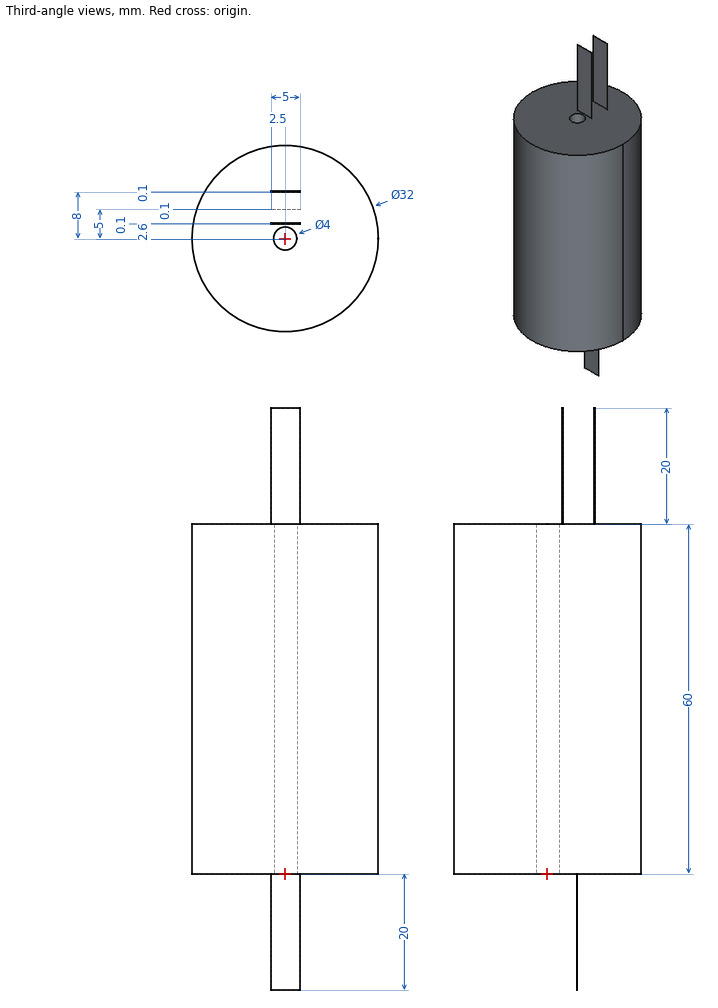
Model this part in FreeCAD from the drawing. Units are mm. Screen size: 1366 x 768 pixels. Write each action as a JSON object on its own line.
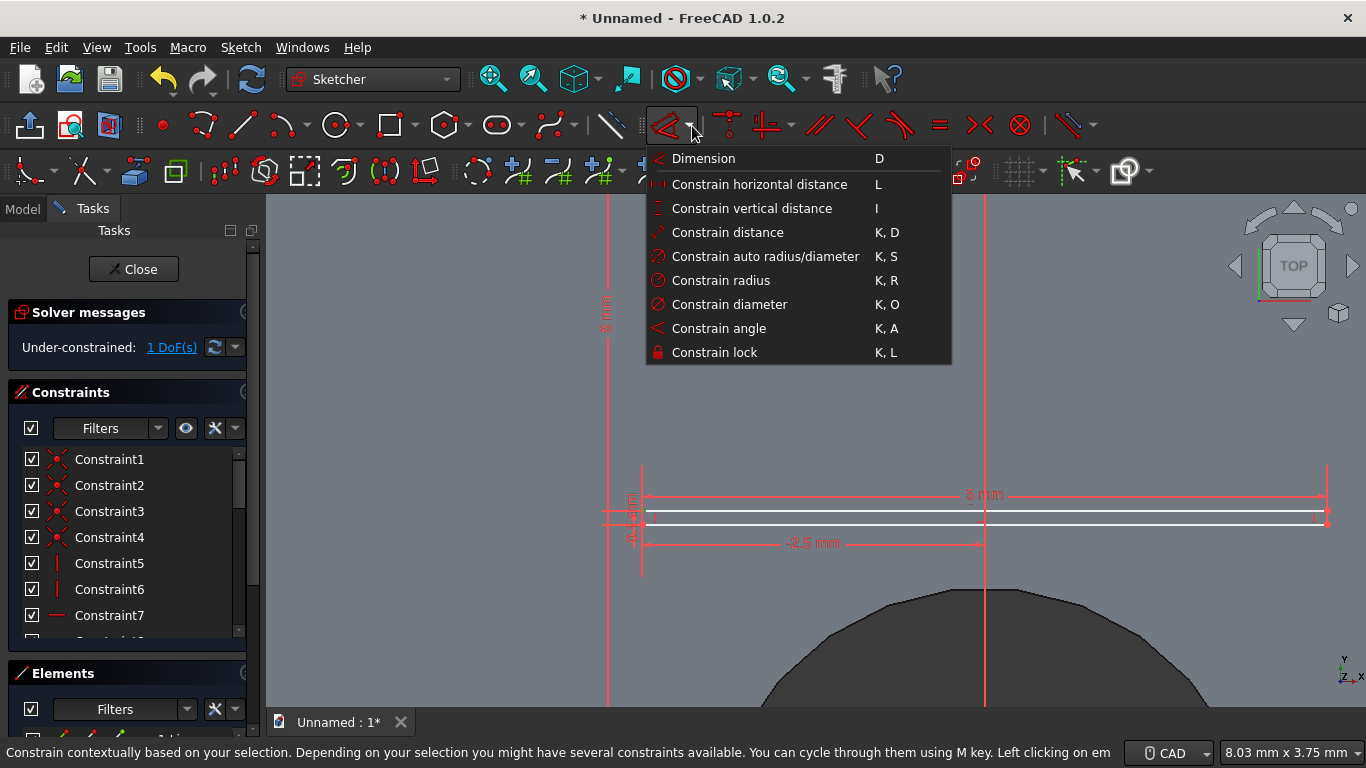
{"action": "left_click", "coordinate": [799, 208]}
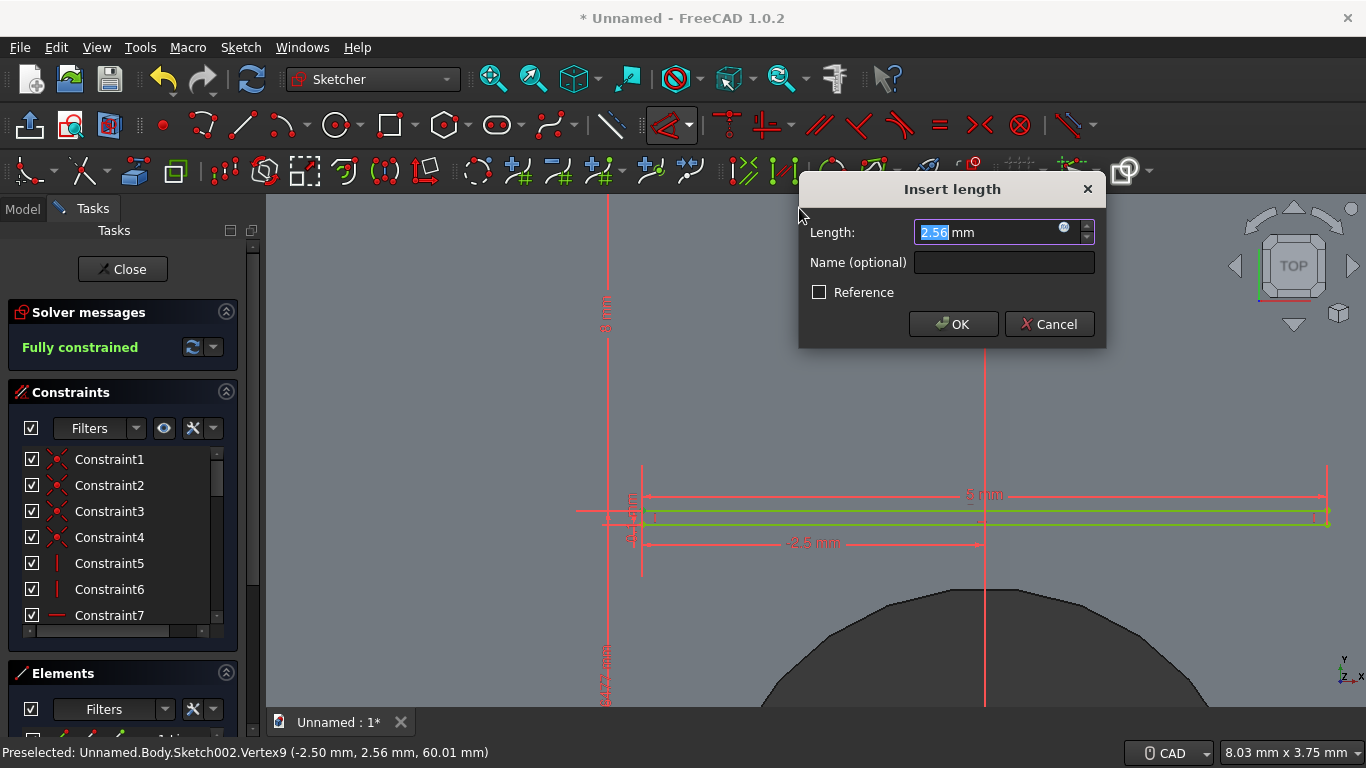
{"action": "type", "text": "2.6"}
{"action": "key", "text": "Return"}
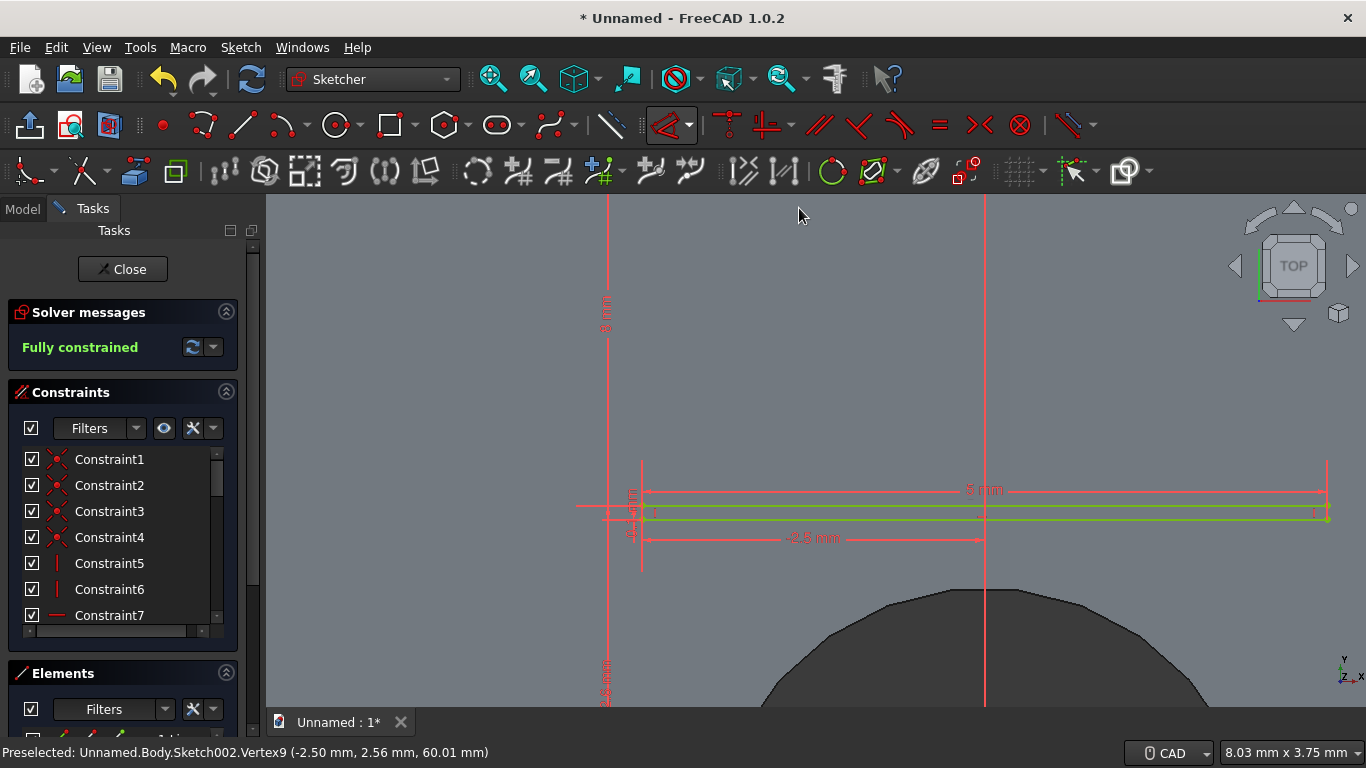
{"action": "left_click", "coordinate": [123, 269]}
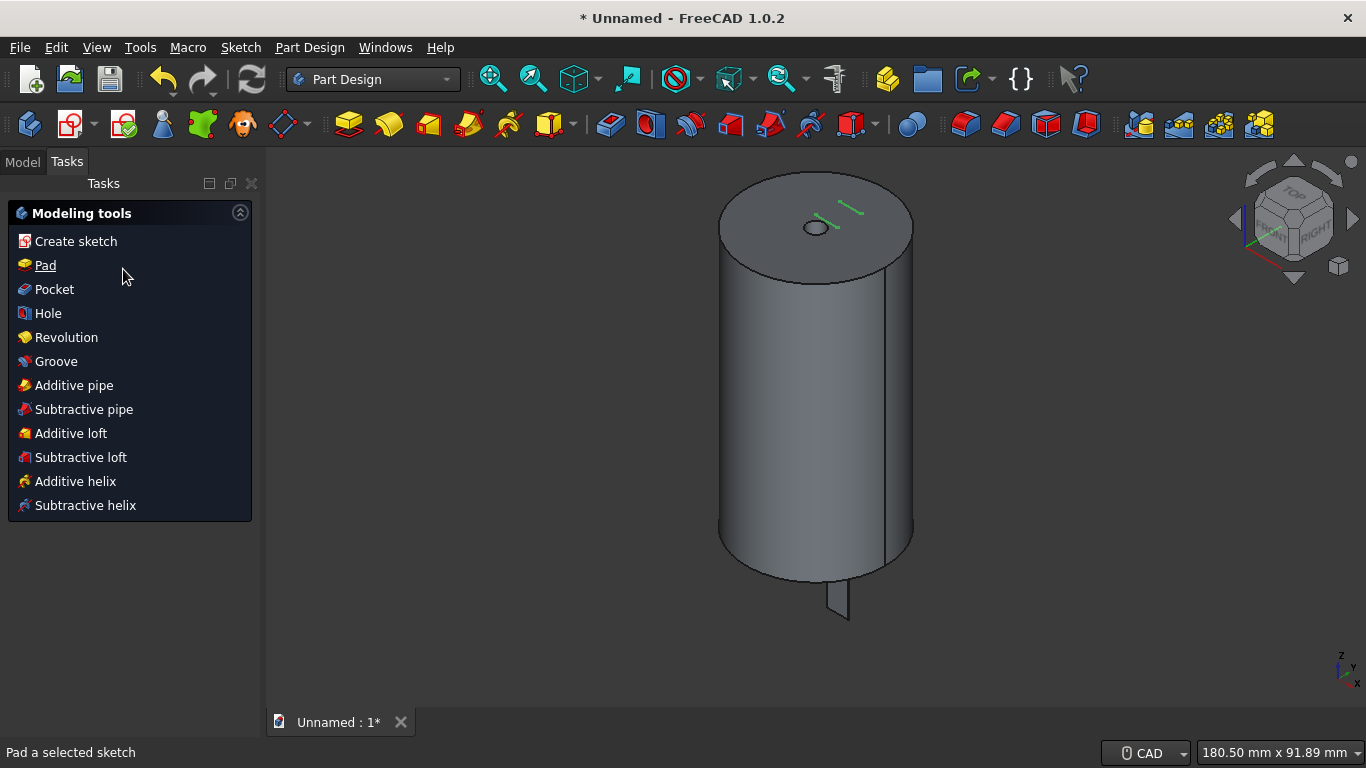
{"action": "left_click", "coordinate": [350, 124]}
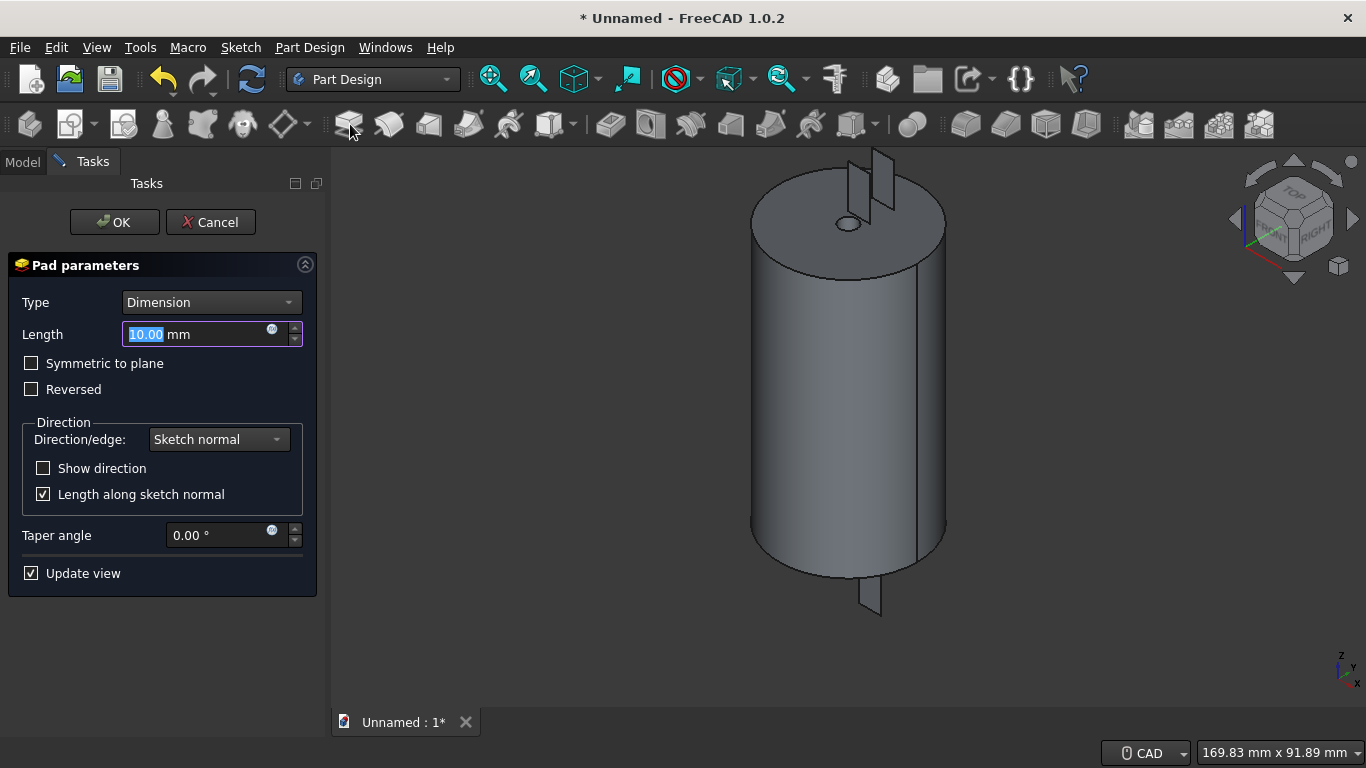
{"action": "type", "text": "20"}
{"action": "key", "text": "Tab"}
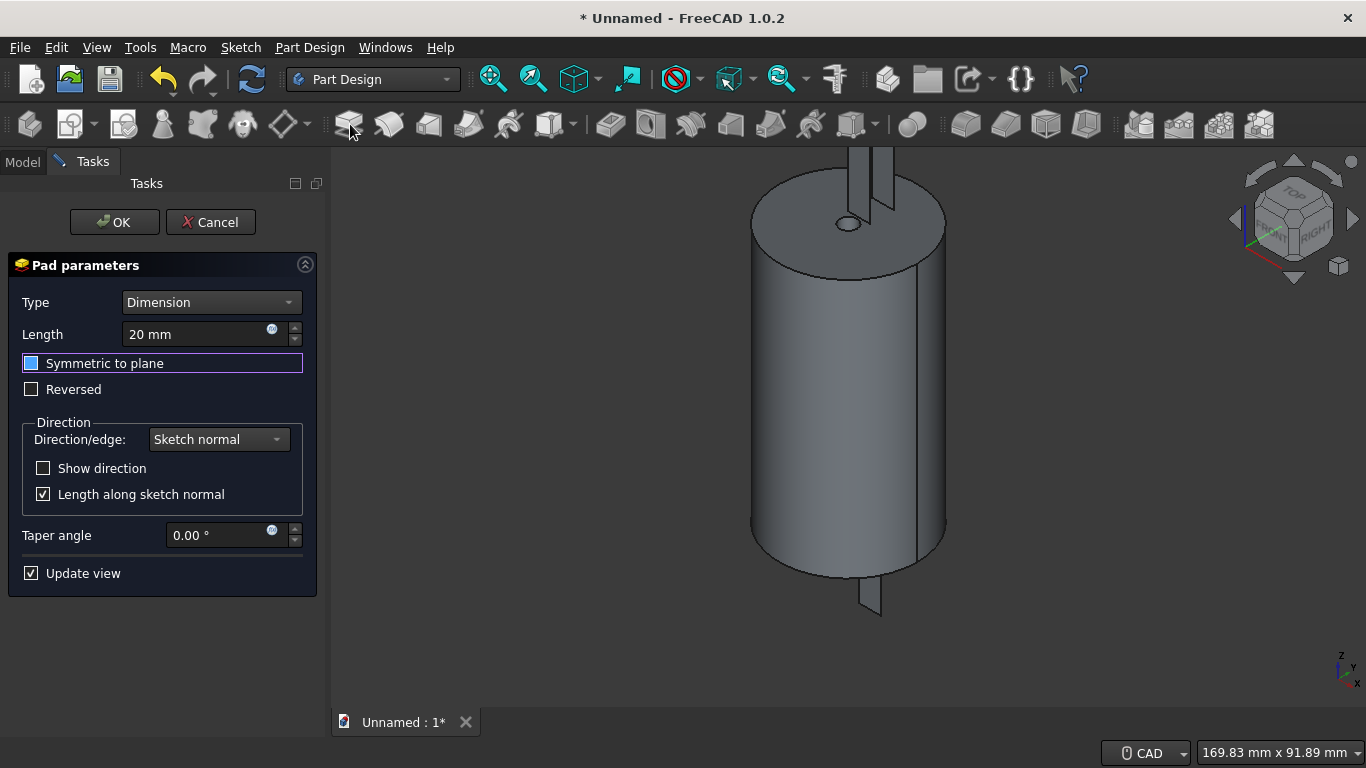
{"action": "left_click", "coordinate": [115, 222]}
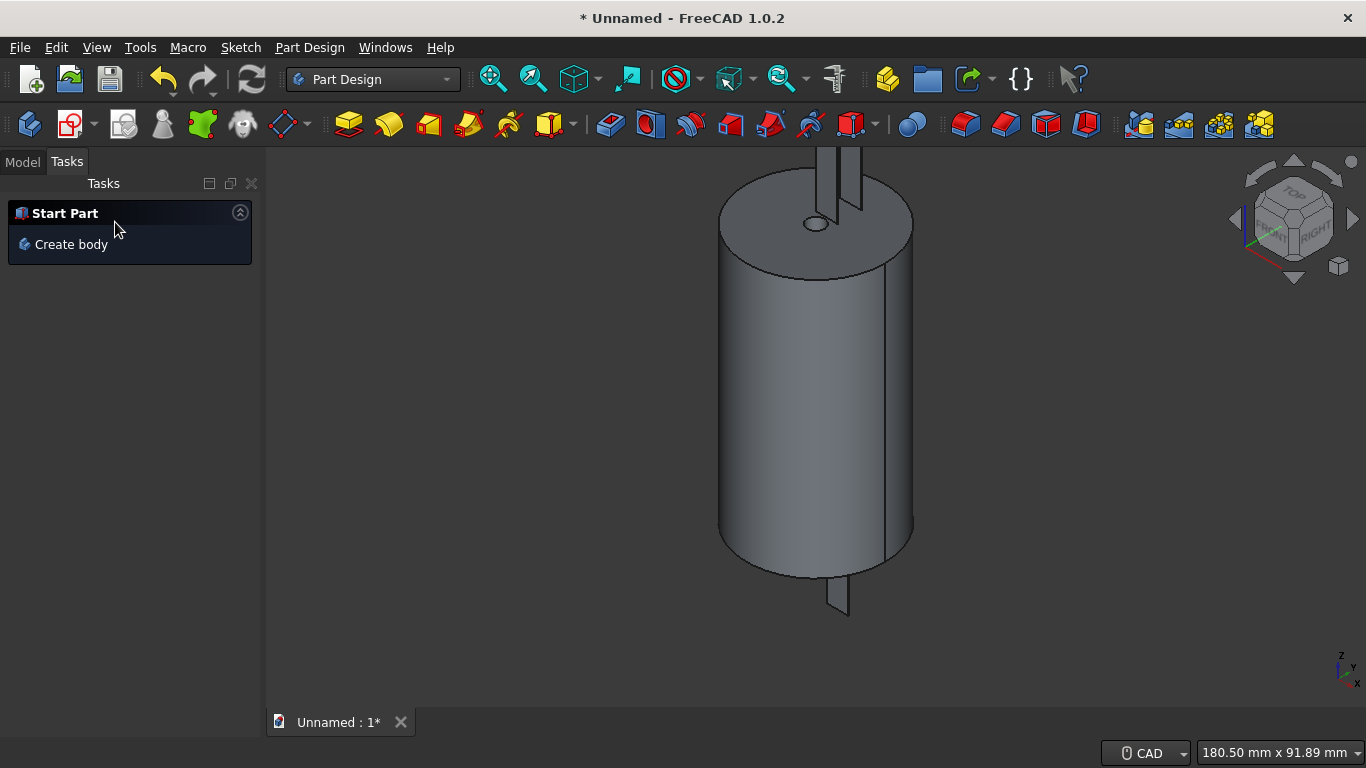
{"action": "left_click", "coordinate": [494, 80]}